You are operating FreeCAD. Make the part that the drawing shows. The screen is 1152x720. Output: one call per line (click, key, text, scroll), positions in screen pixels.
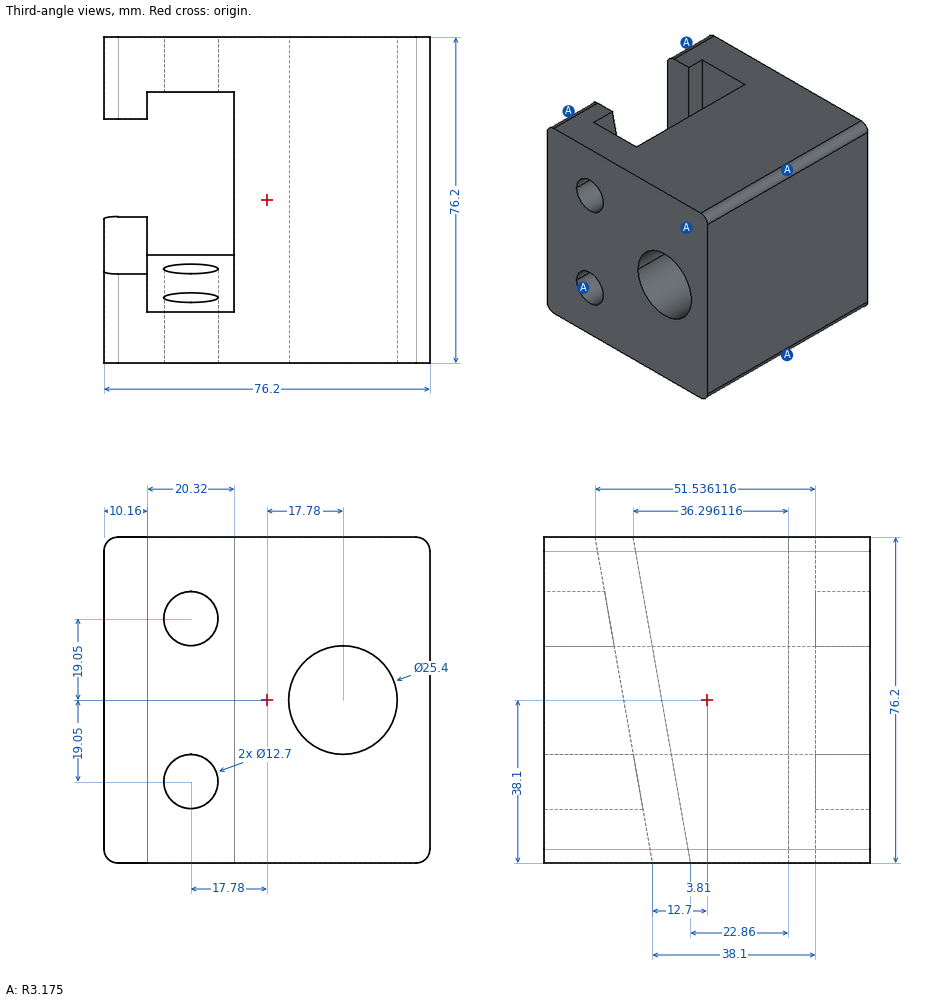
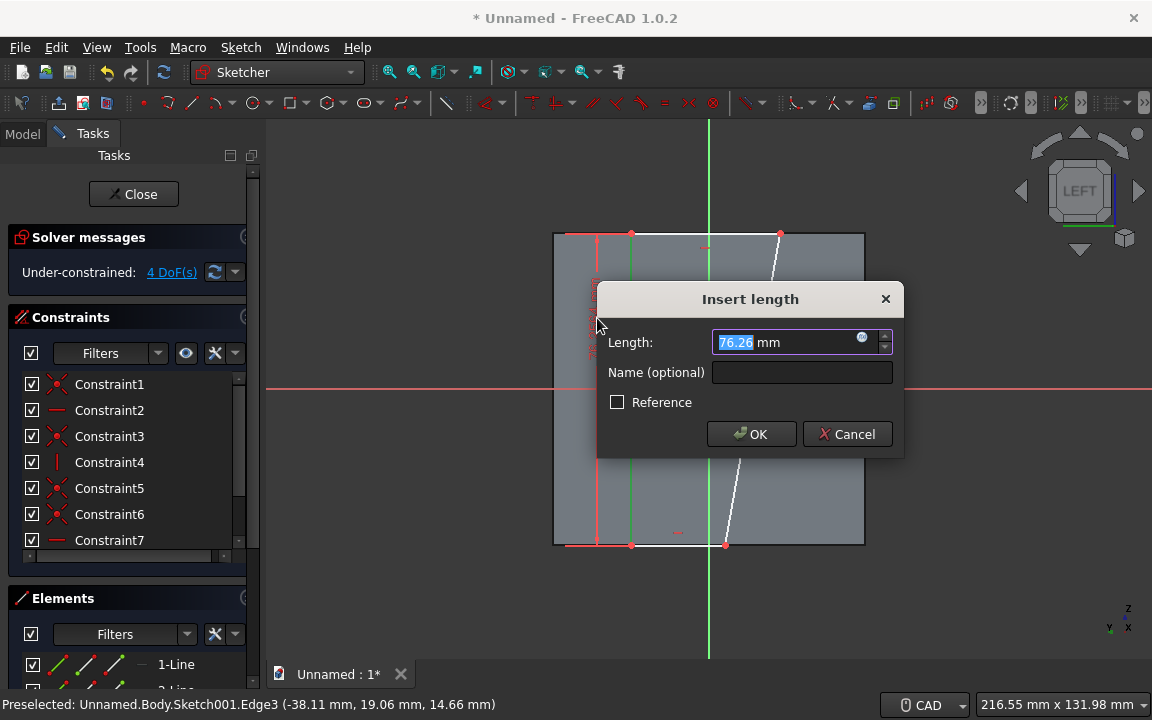
text(76.2)
key(Return)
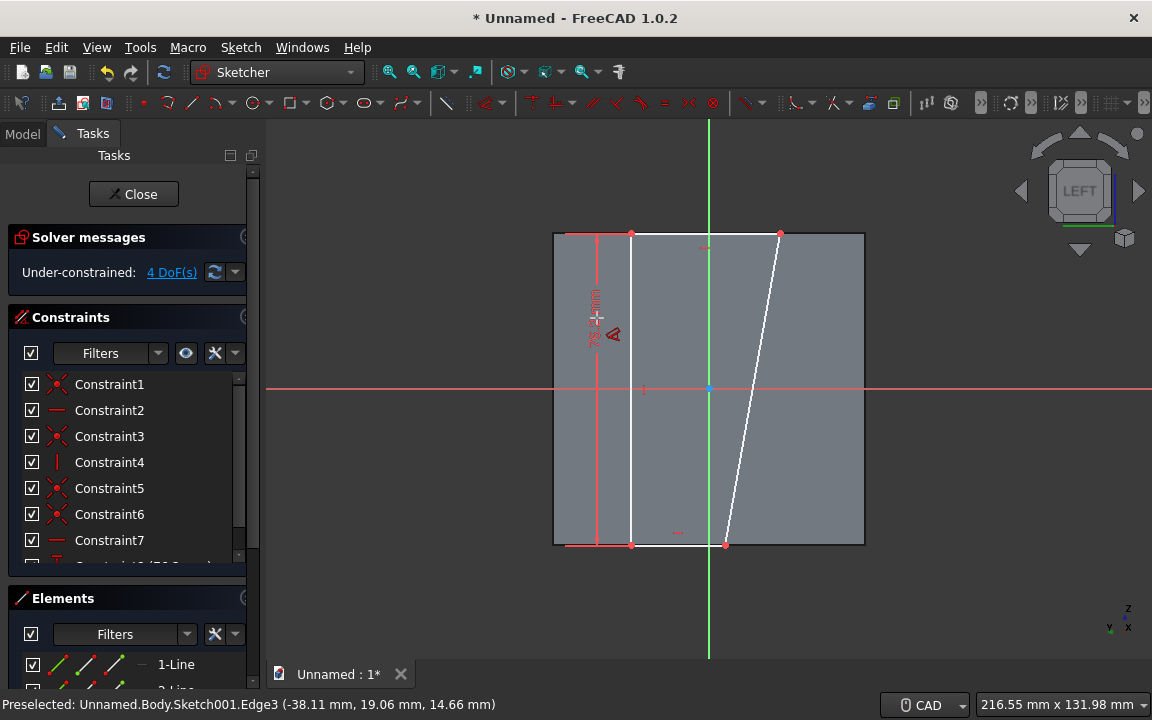
click(659, 546)
click(678, 580)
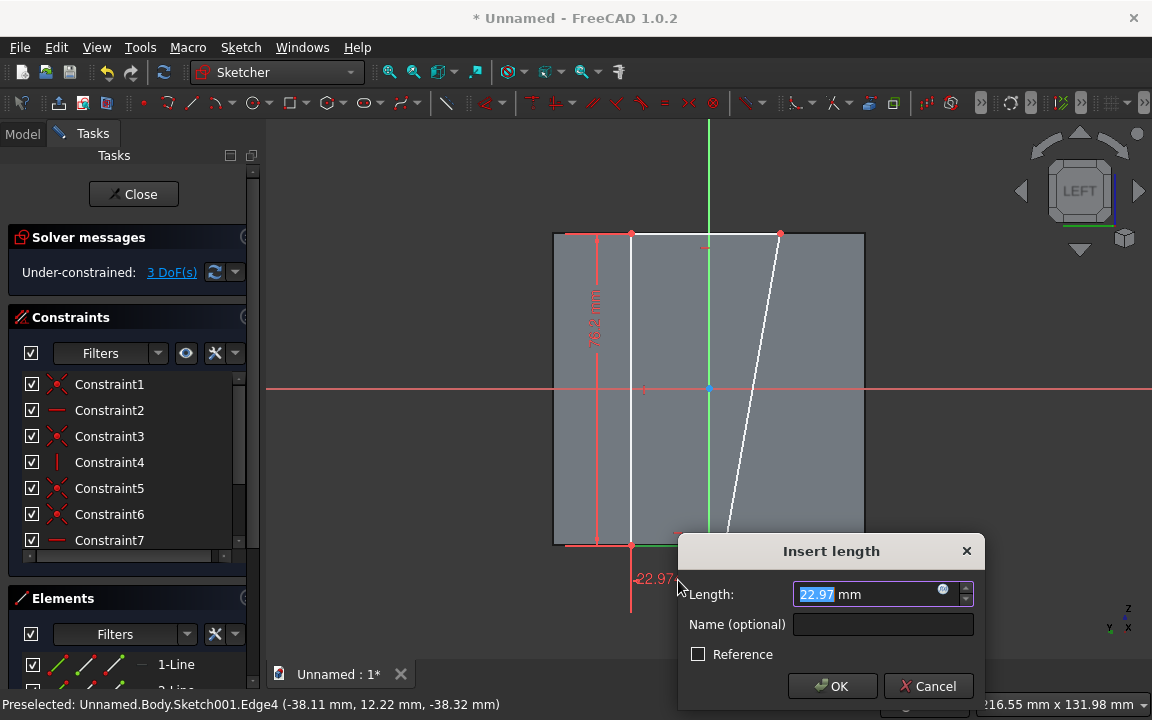
text(22.86)
key(Return)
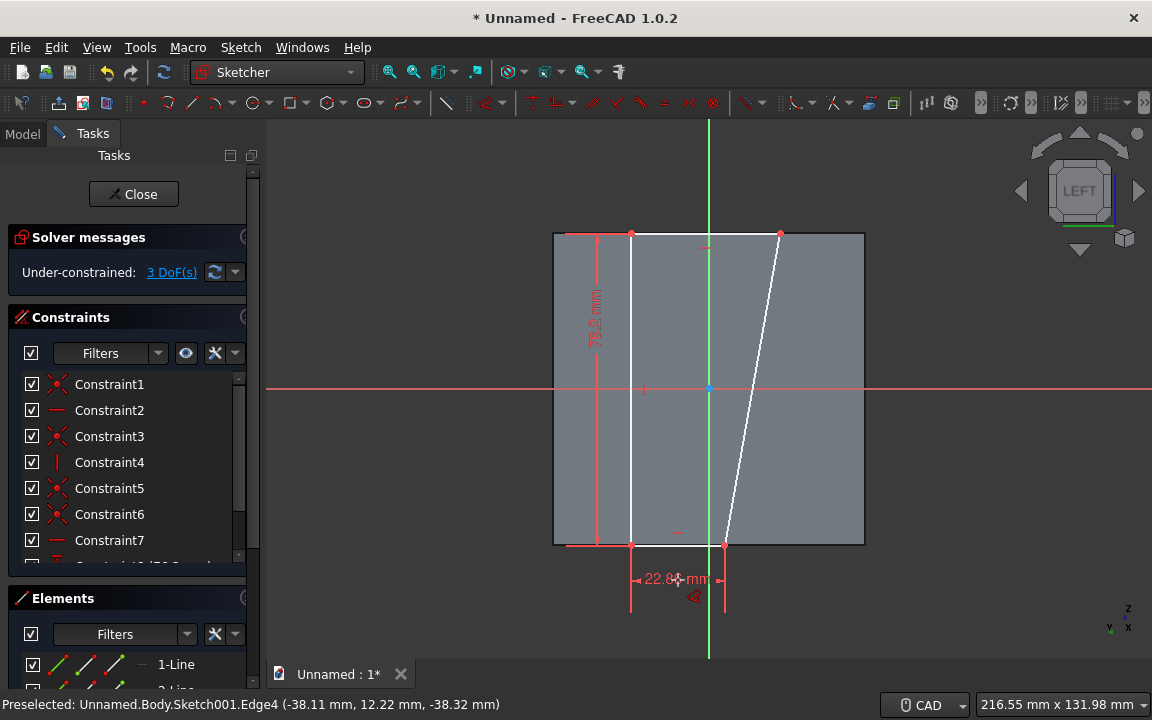
scroll(725, 546, up, 5)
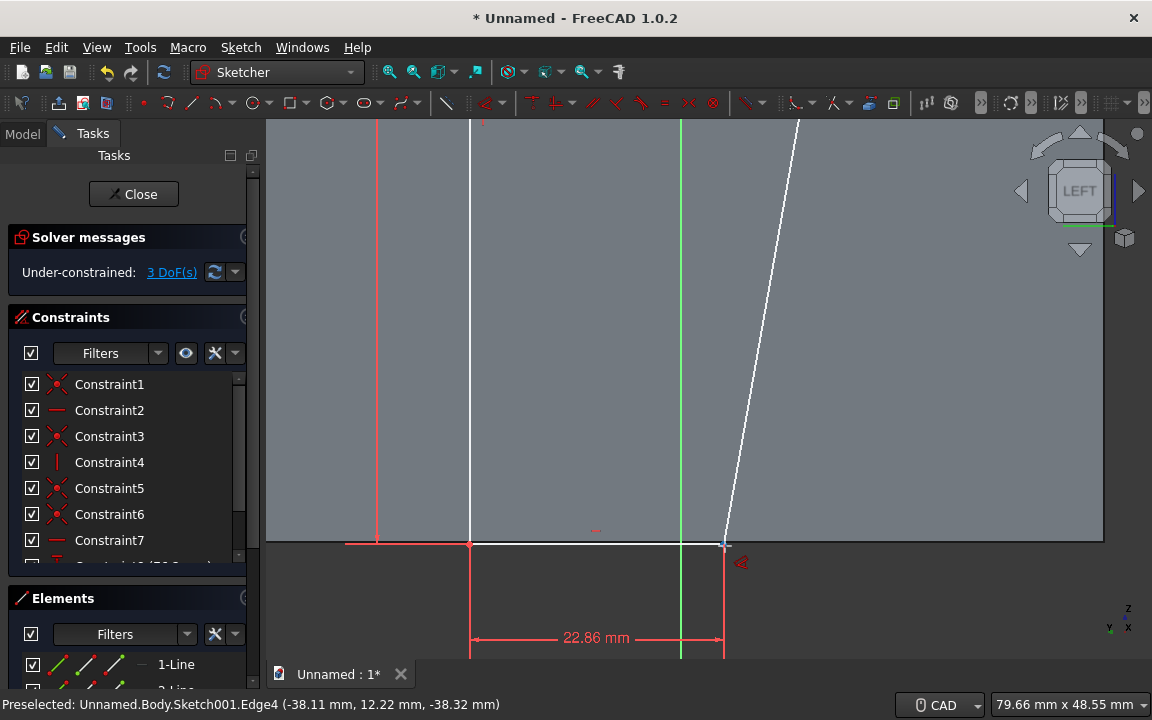
click(724, 544)
click(702, 578)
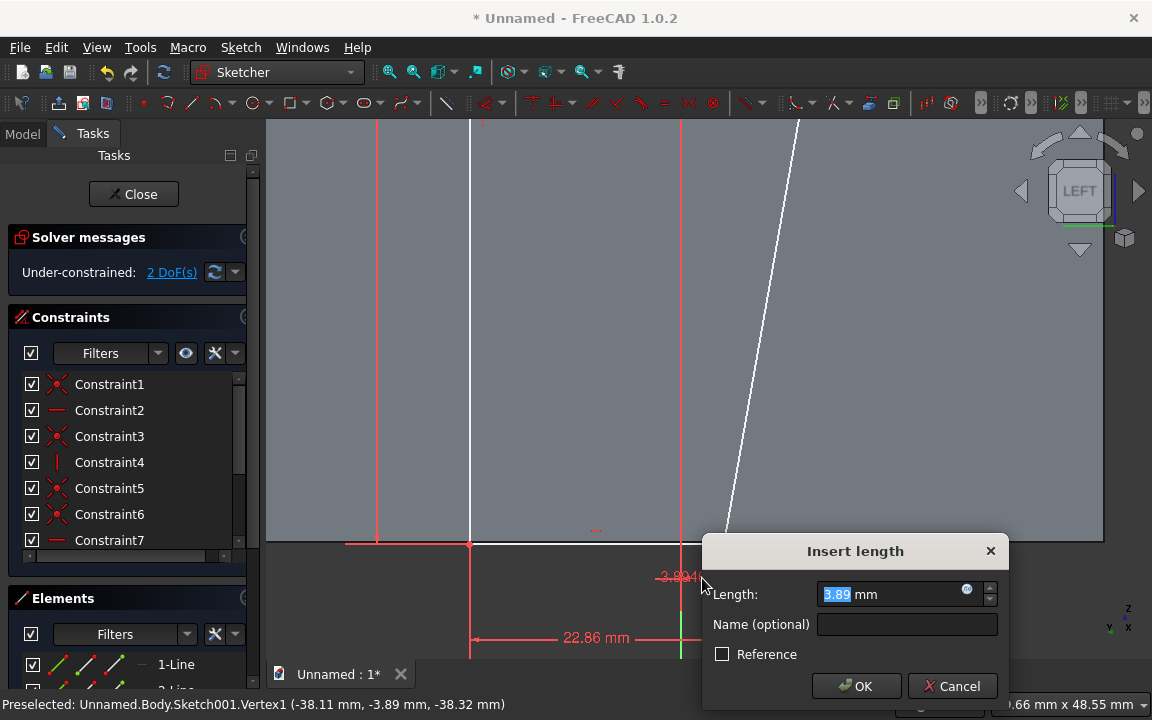
text(3.81)
key(Return)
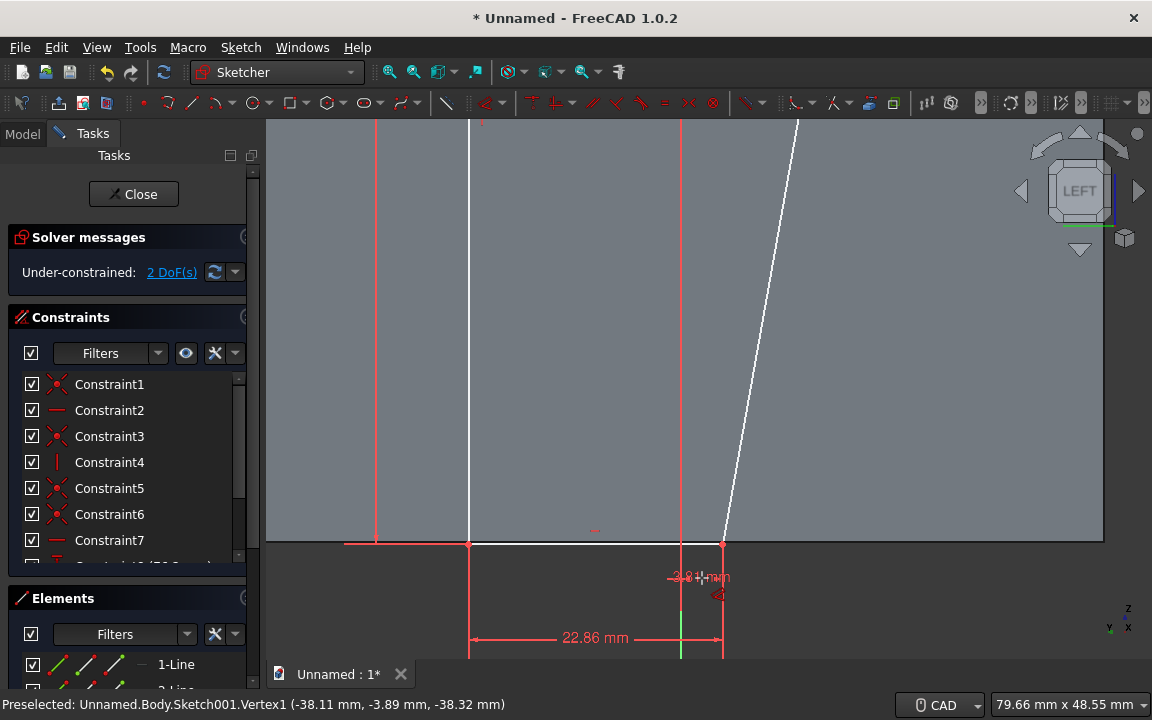
click(723, 544)
click(757, 254)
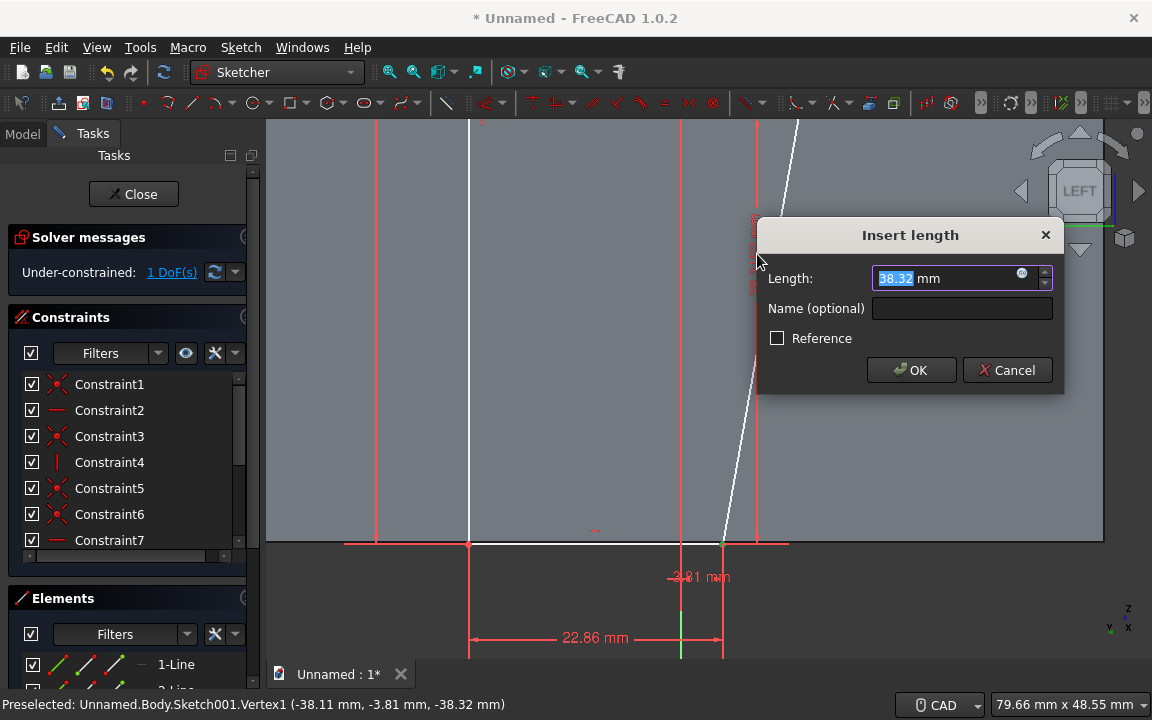
text(38.1)
key(Return)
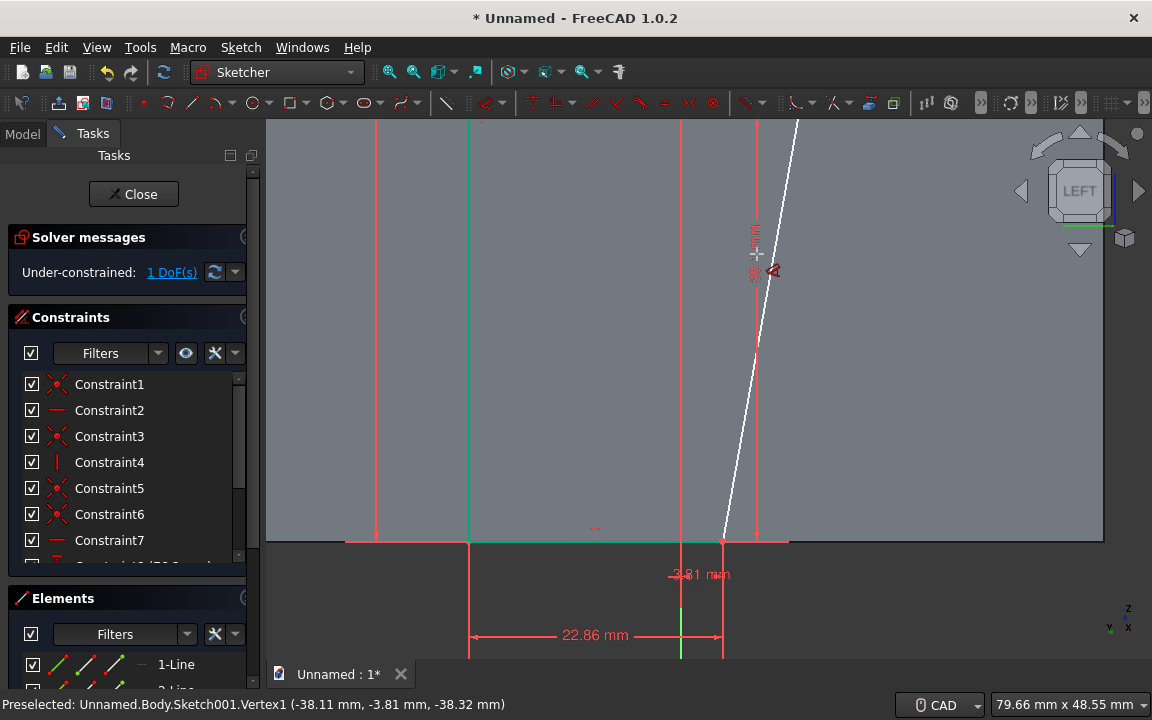
scroll(623, 547, down, 5)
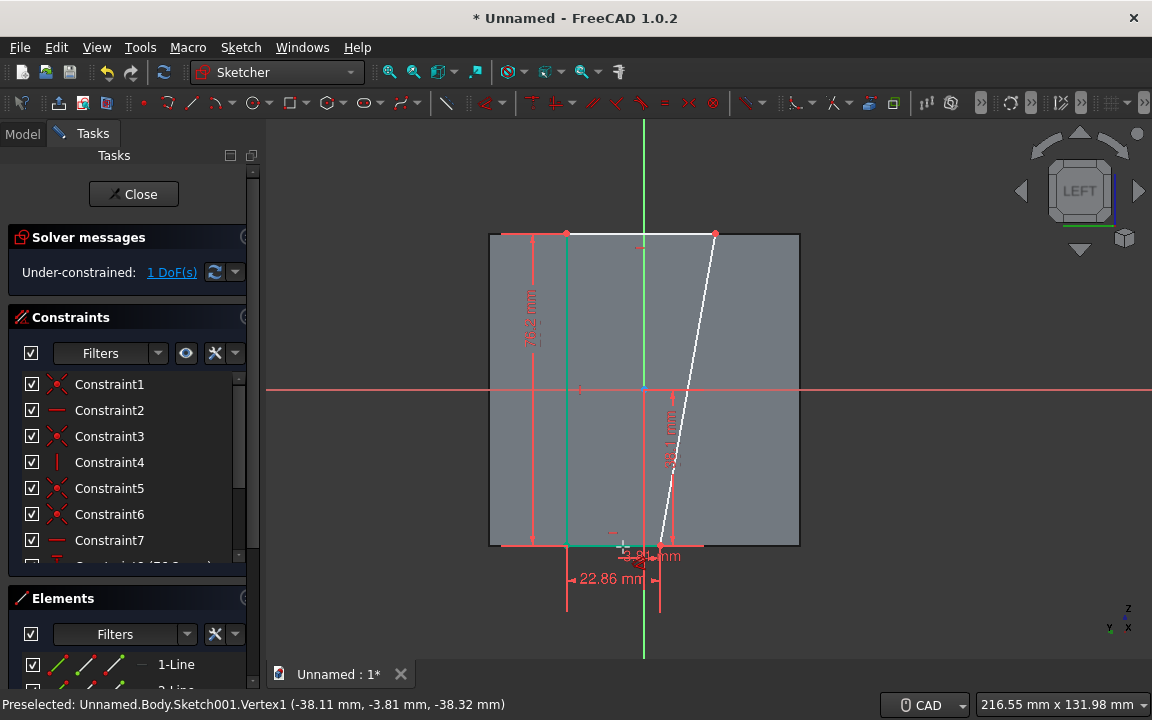
click(671, 234)
click(607, 200)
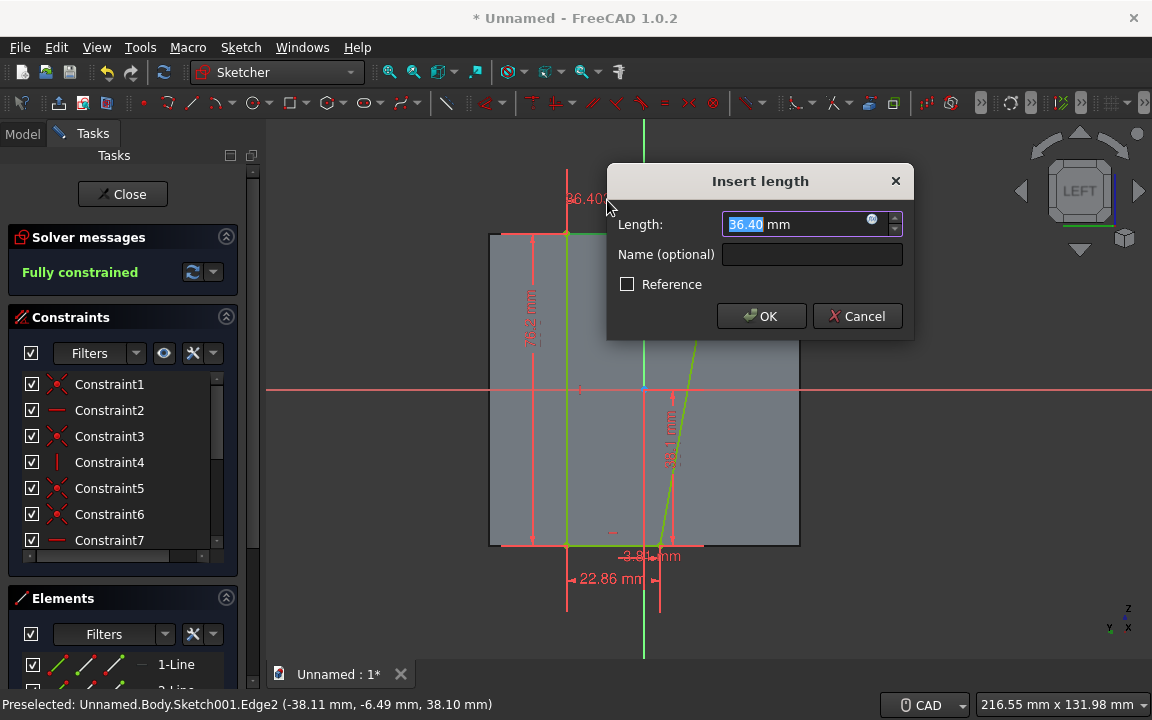
text(36.296116)
key(Return)
key(Escape)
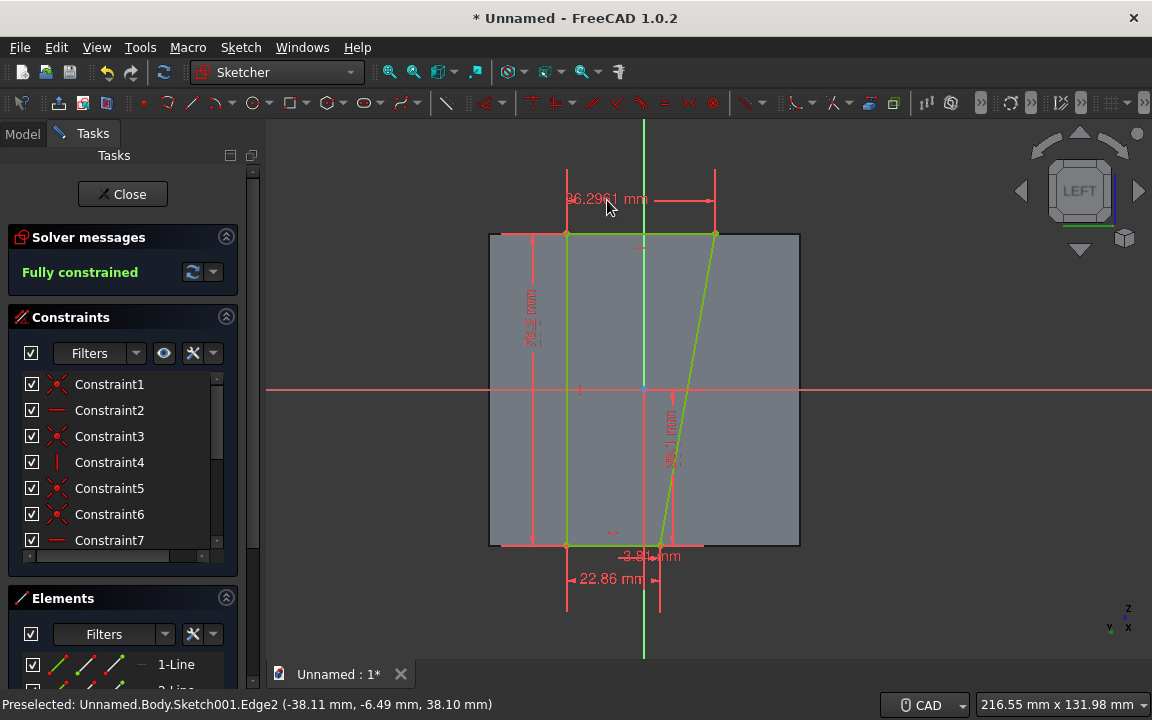
click(123, 194)